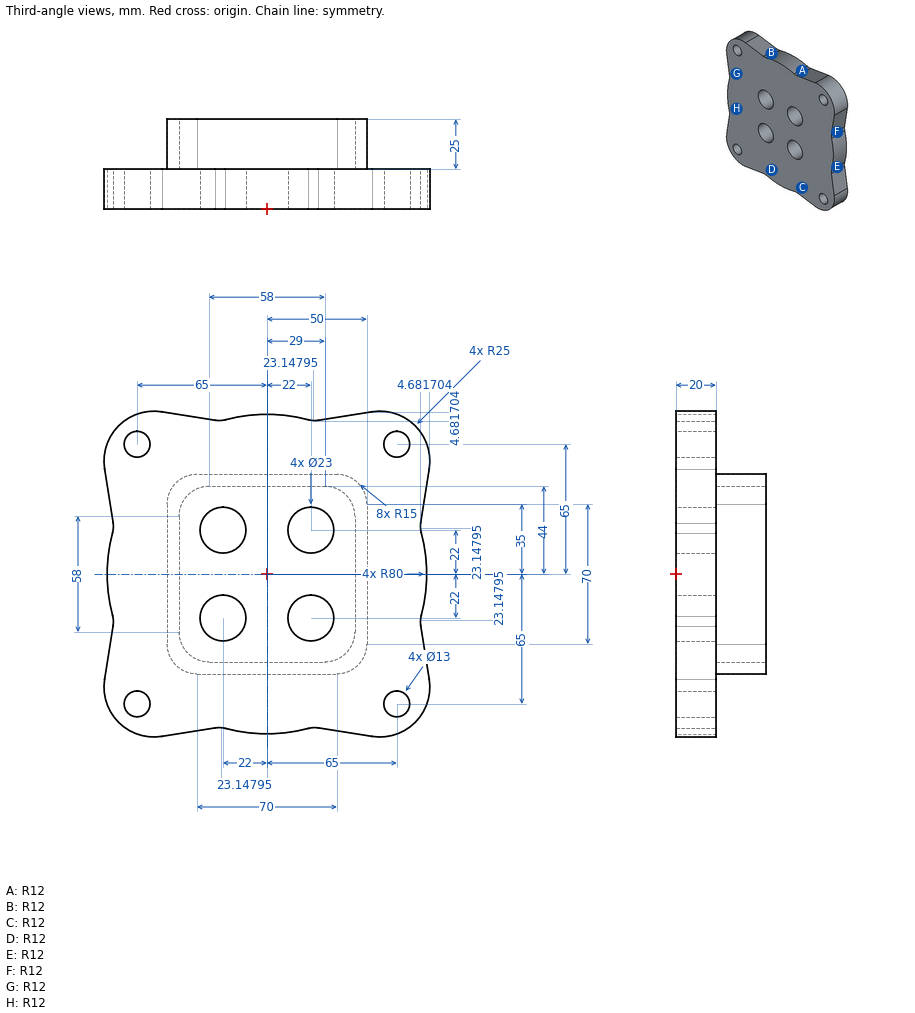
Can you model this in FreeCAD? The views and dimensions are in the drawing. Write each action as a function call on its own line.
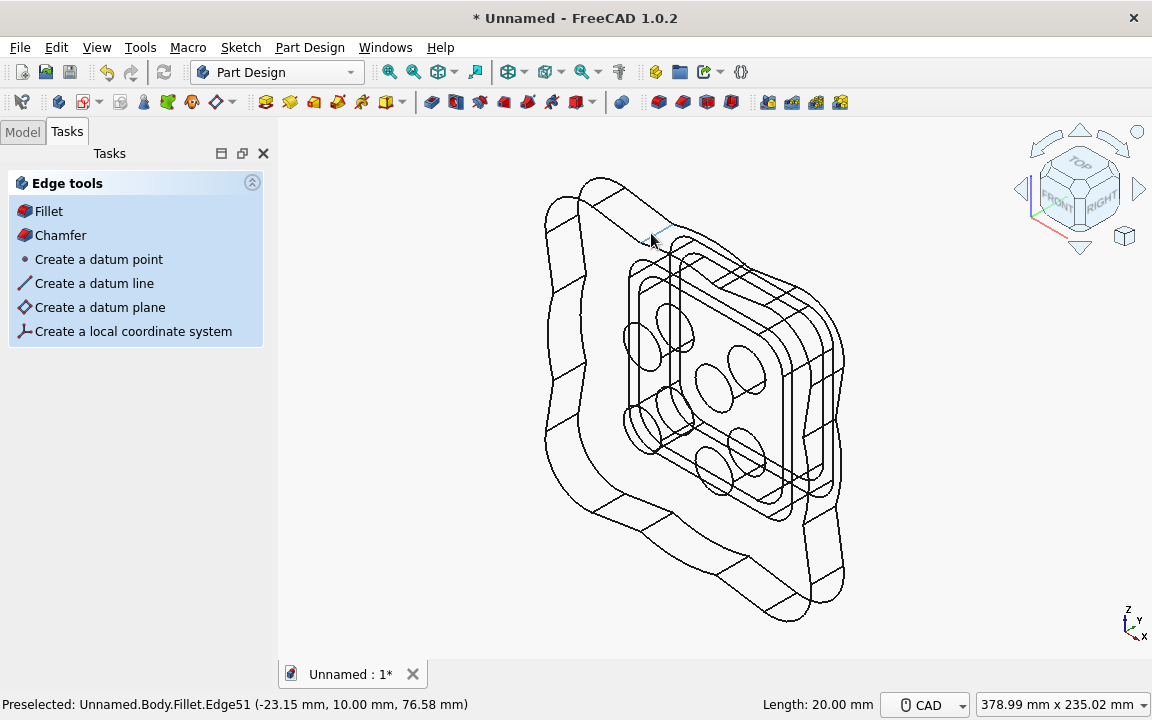
key(v)
key(1)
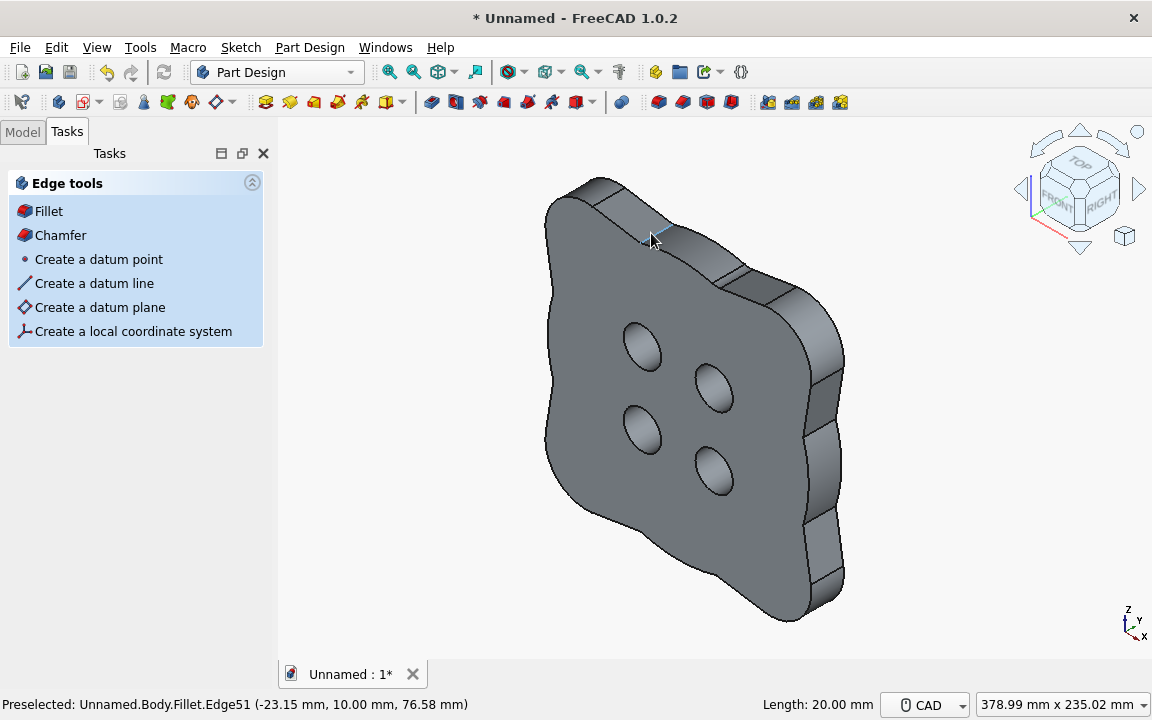
click(660, 102)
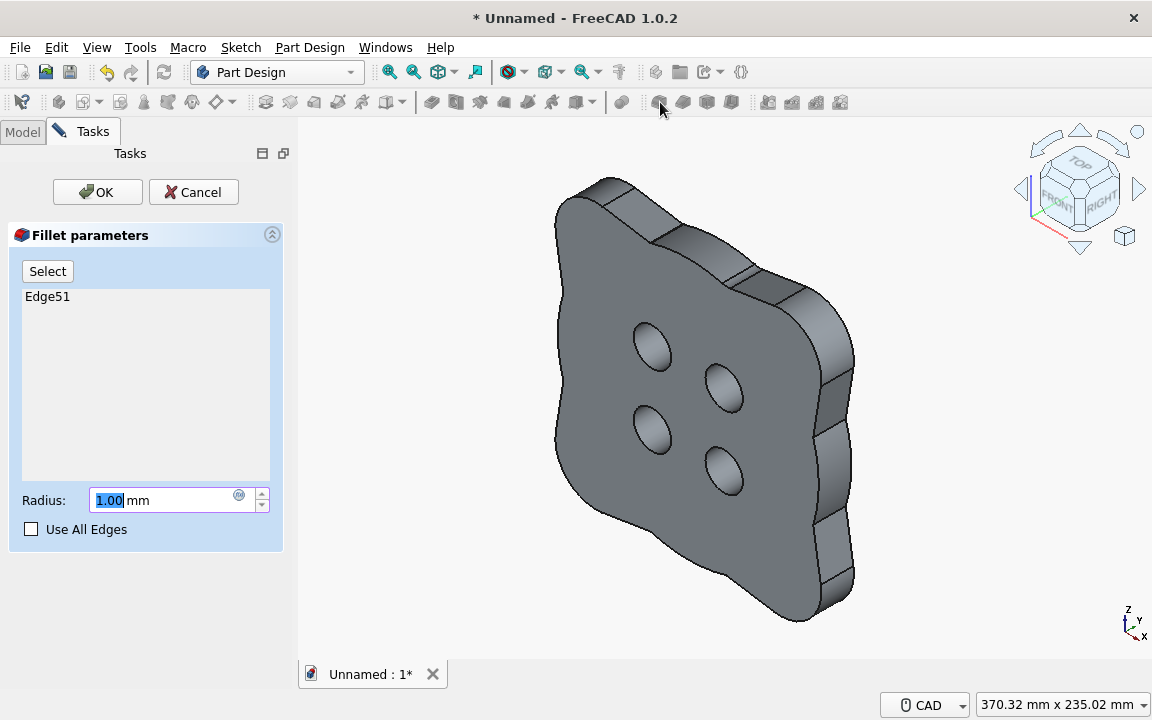
text(12)
key(Tab)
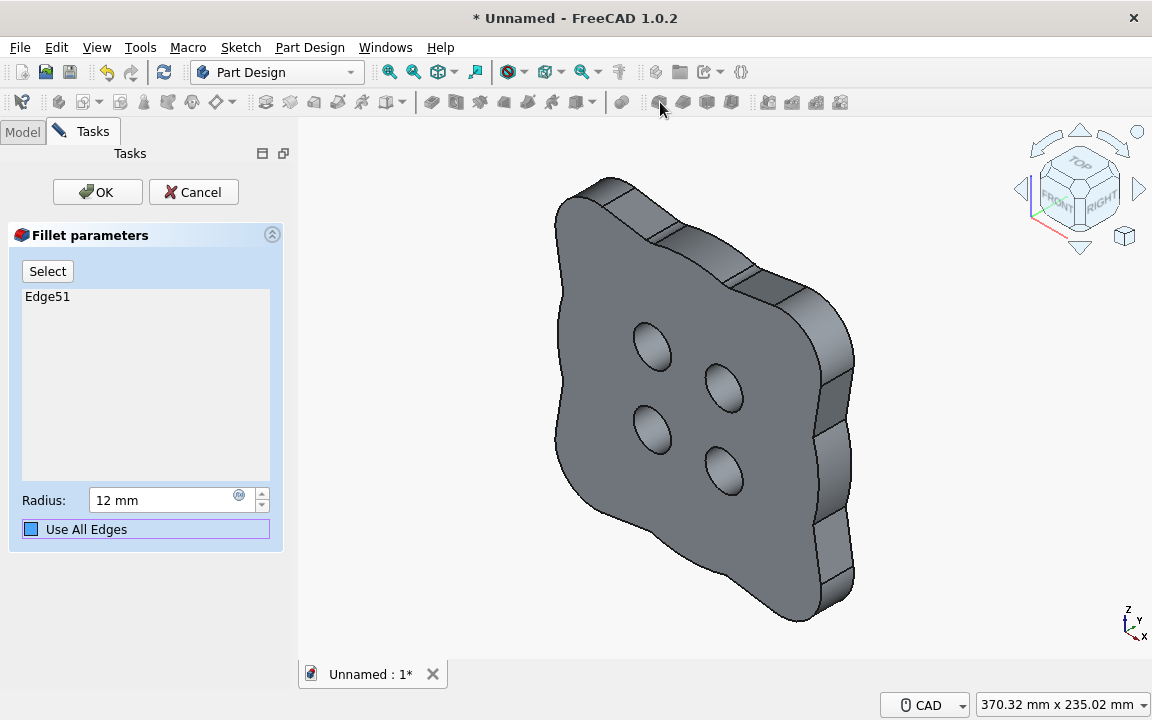
click(98, 192)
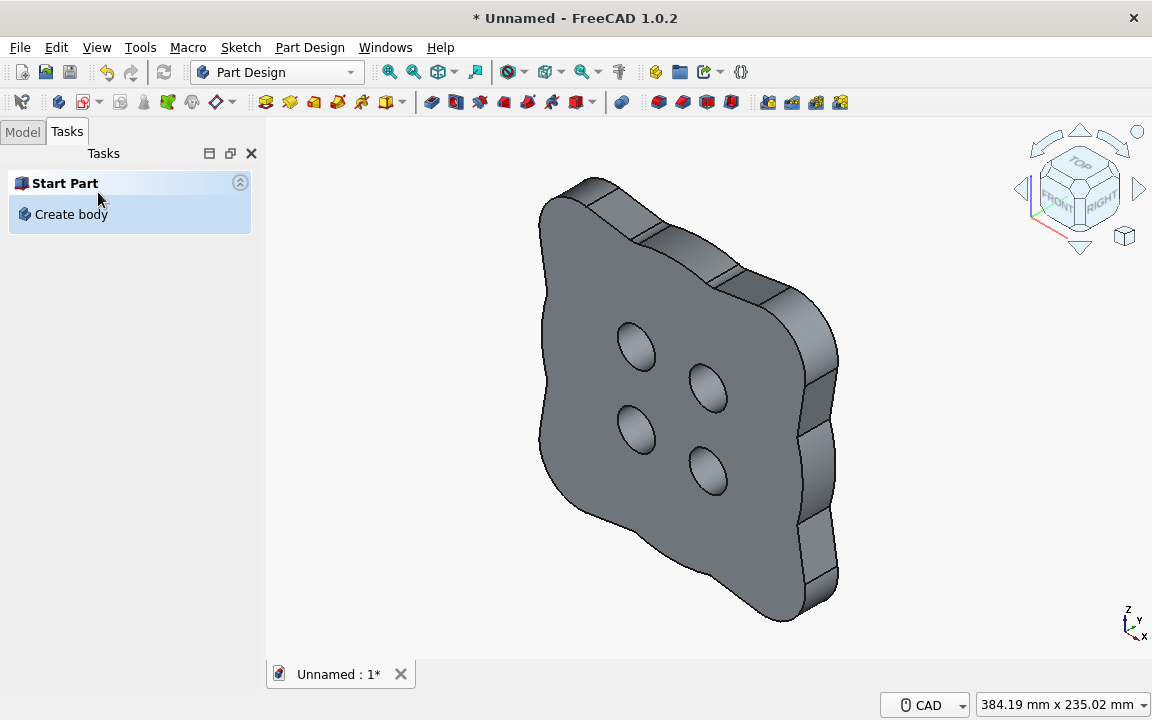
key(2)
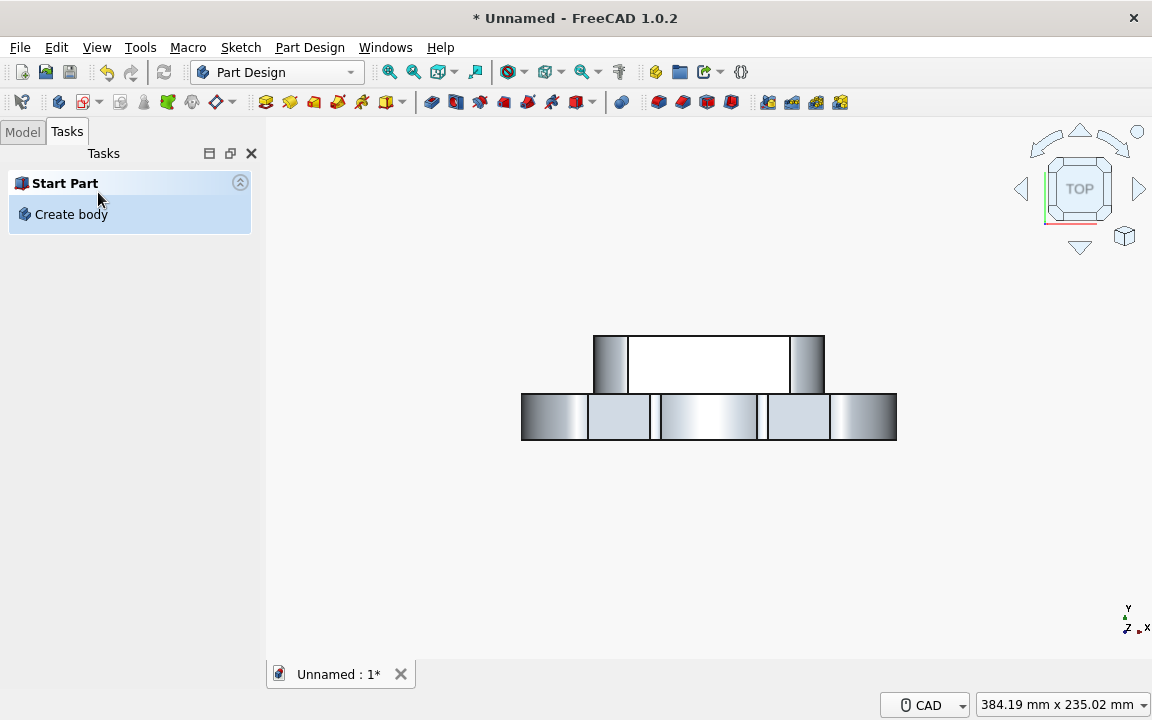
click(390, 72)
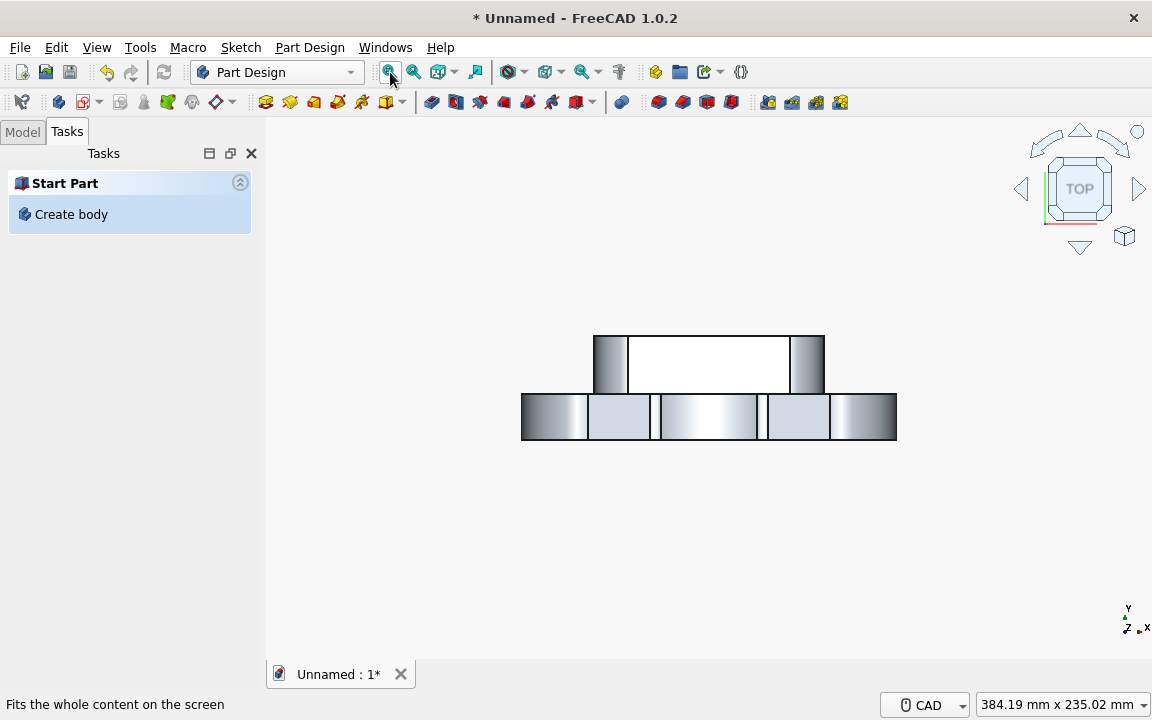
key(0)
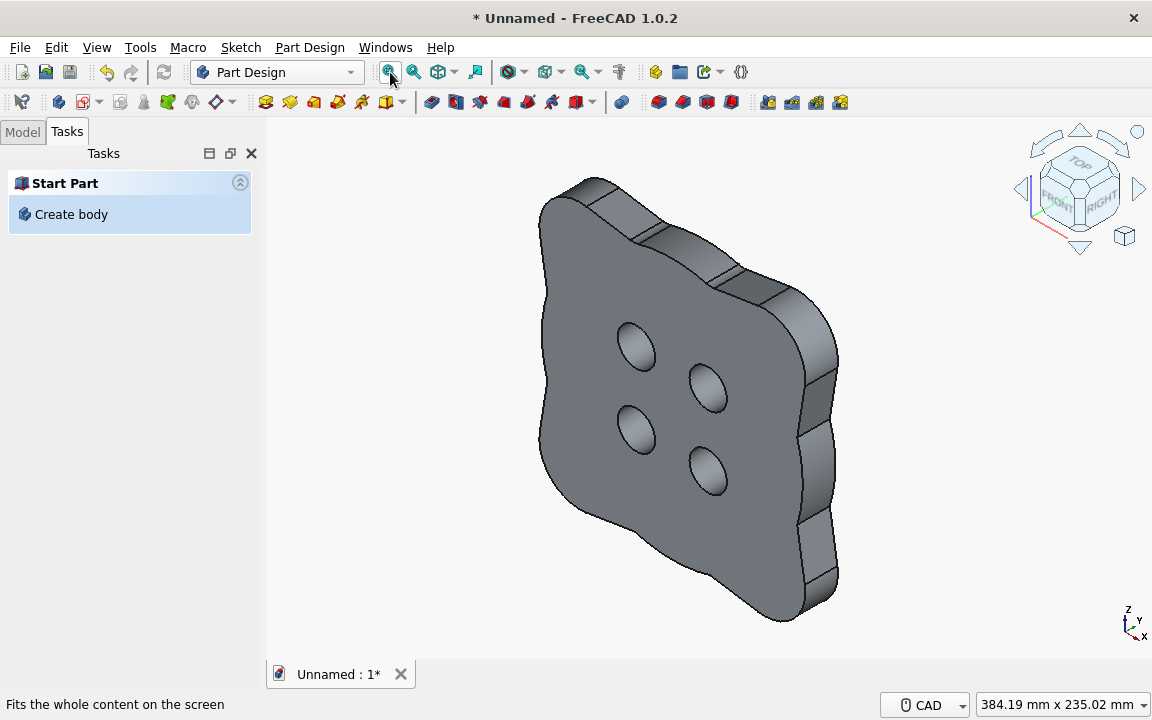
key(1)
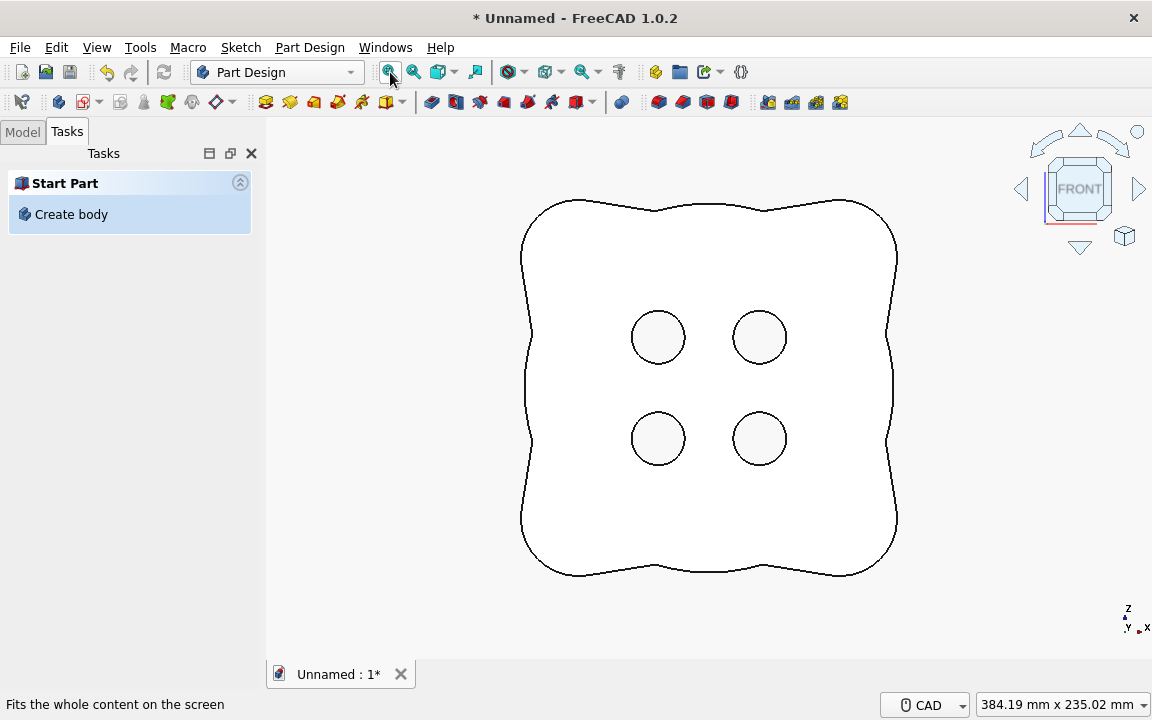
key(3)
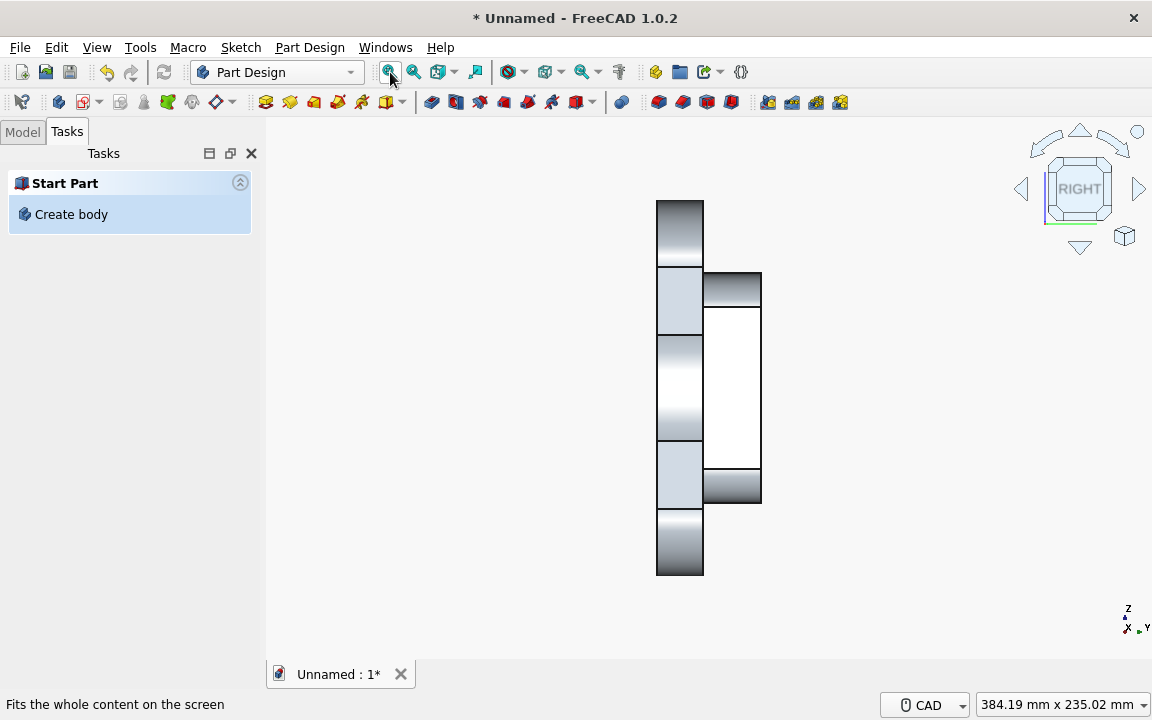
key(5)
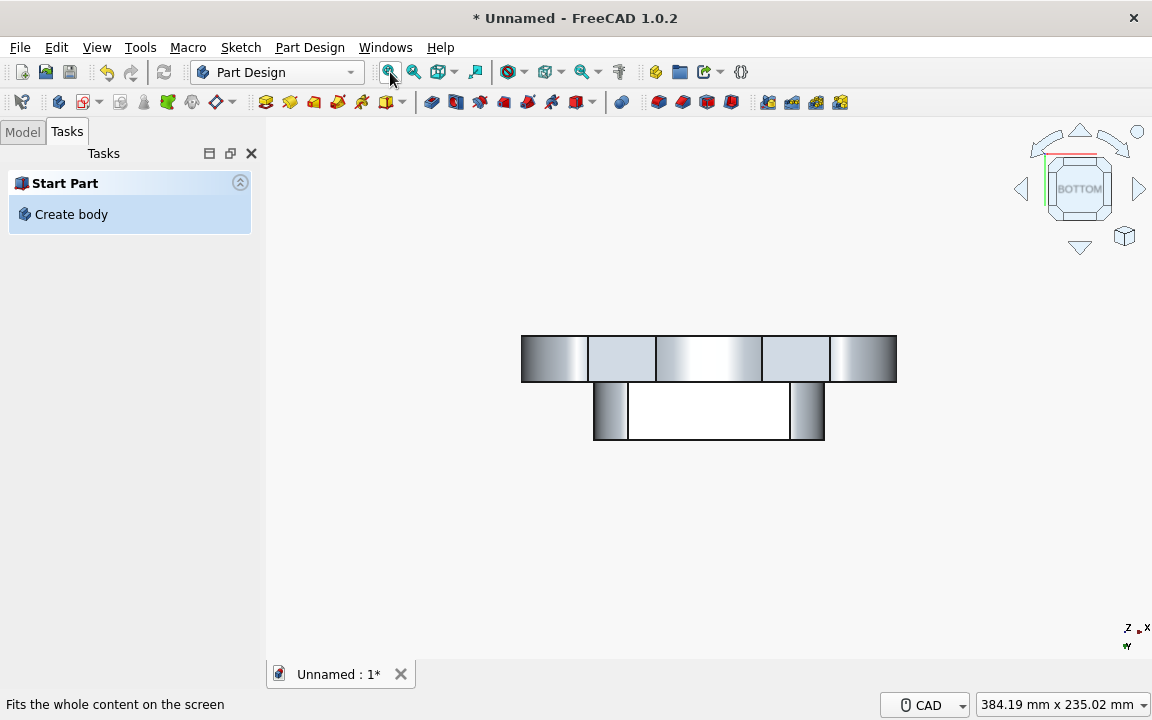
click(390, 72)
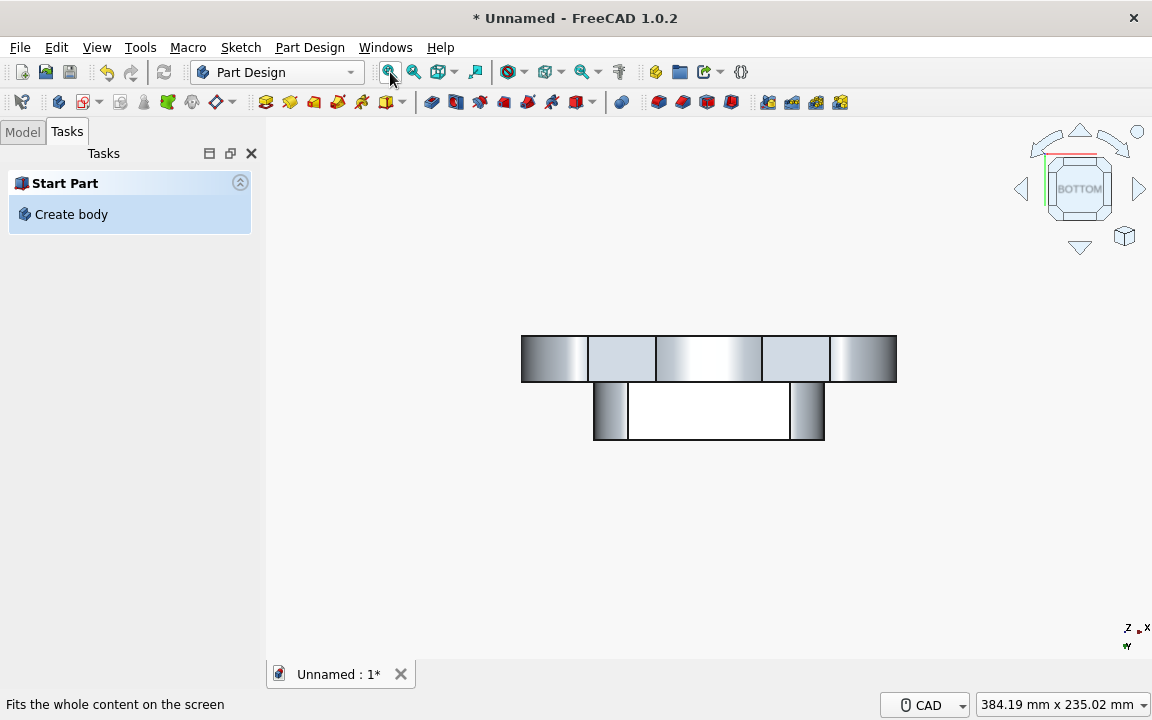
key(4)